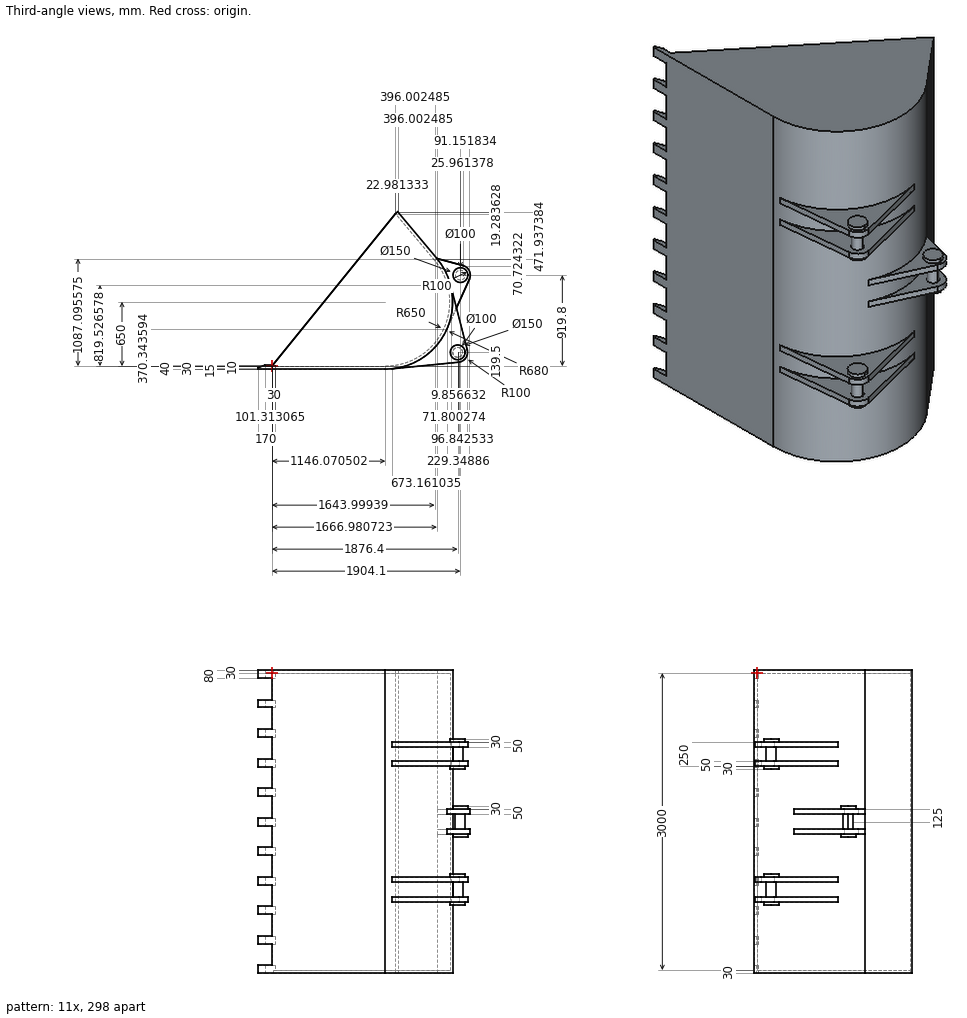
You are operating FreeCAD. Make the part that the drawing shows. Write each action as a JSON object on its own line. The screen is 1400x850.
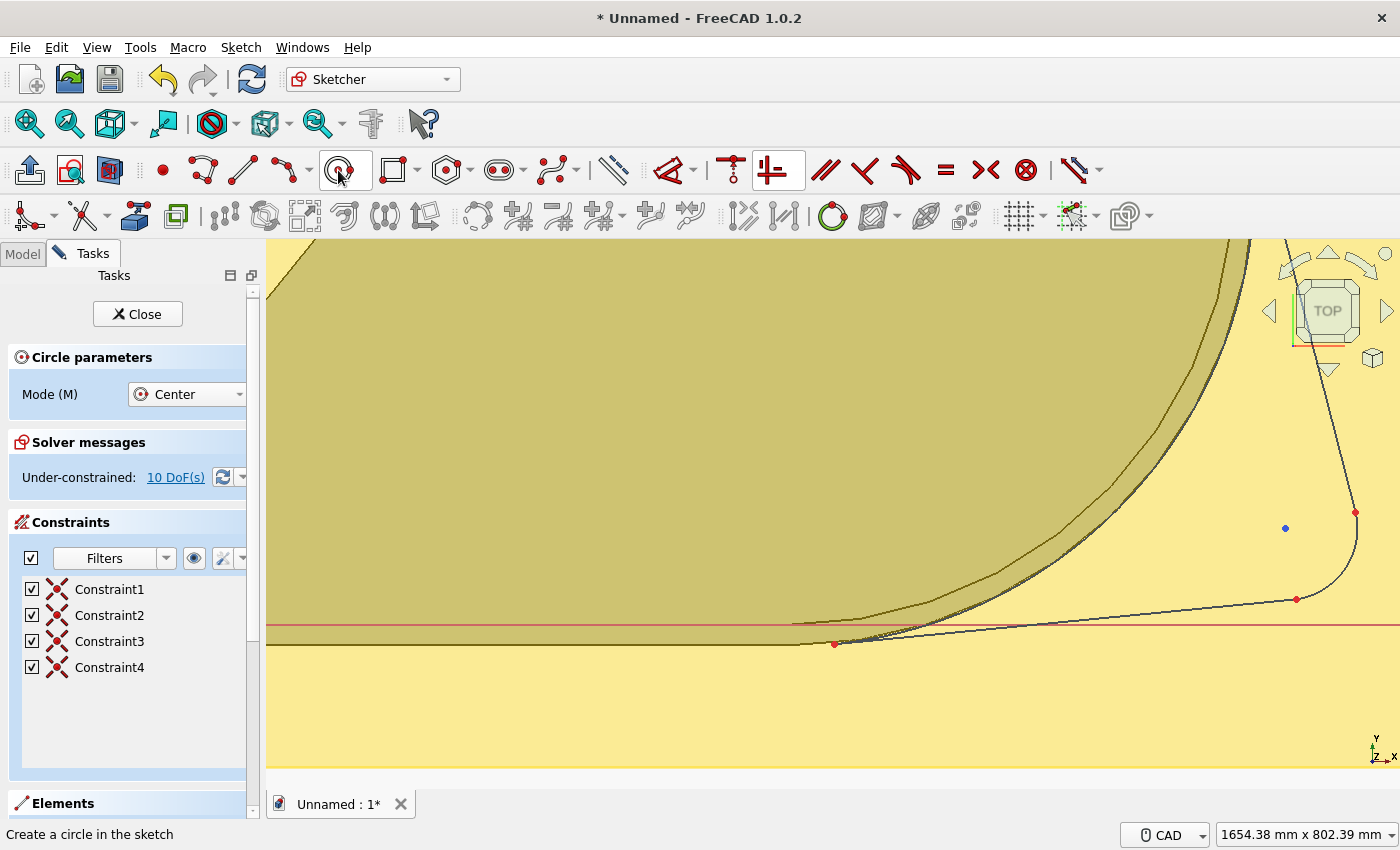
{"action": "scroll", "coordinate": [834, 645], "scroll_direction": "down", "scroll_amount": 4}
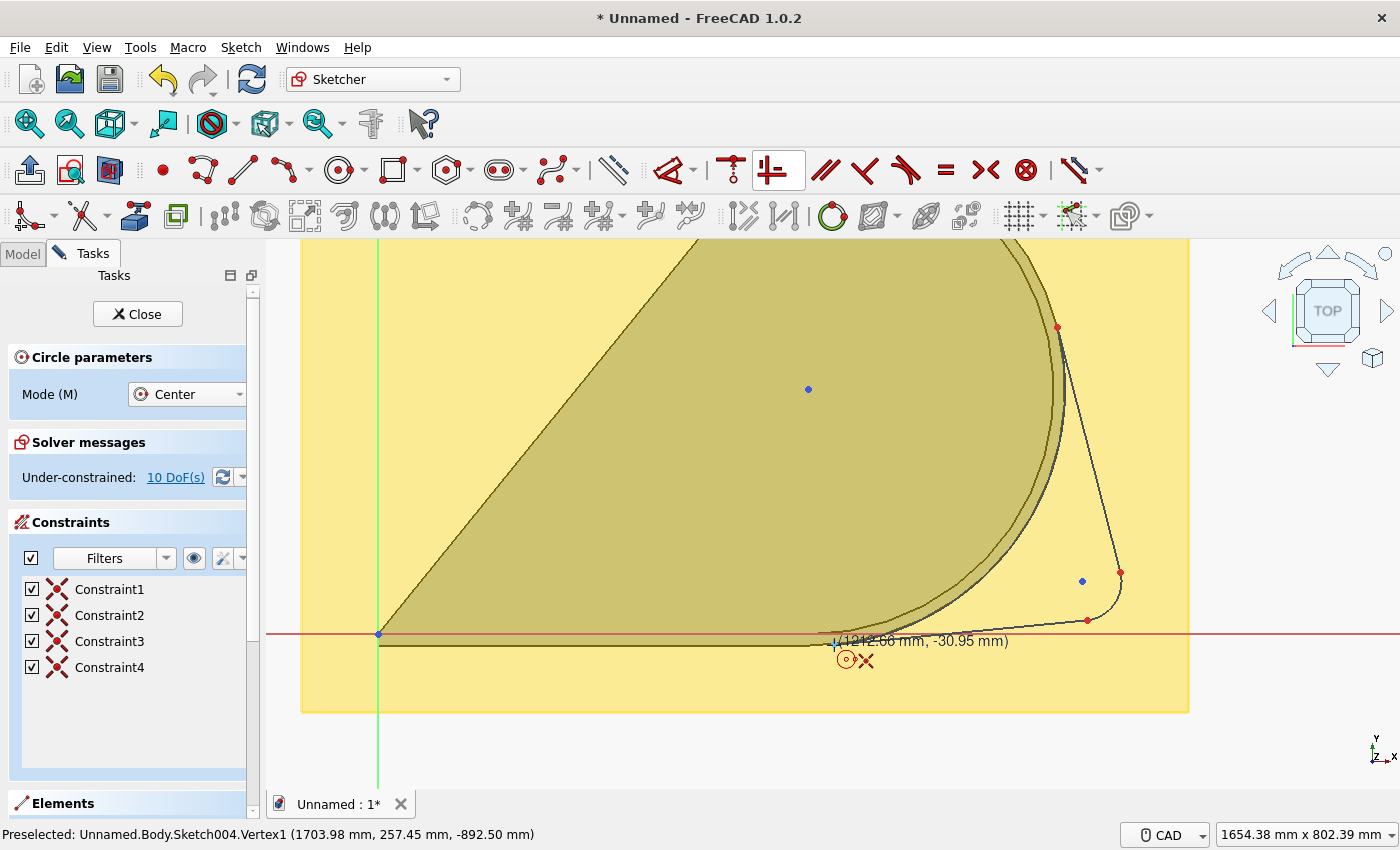
{"action": "scroll", "coordinate": [1039, 593], "scroll_direction": "up", "scroll_amount": 2}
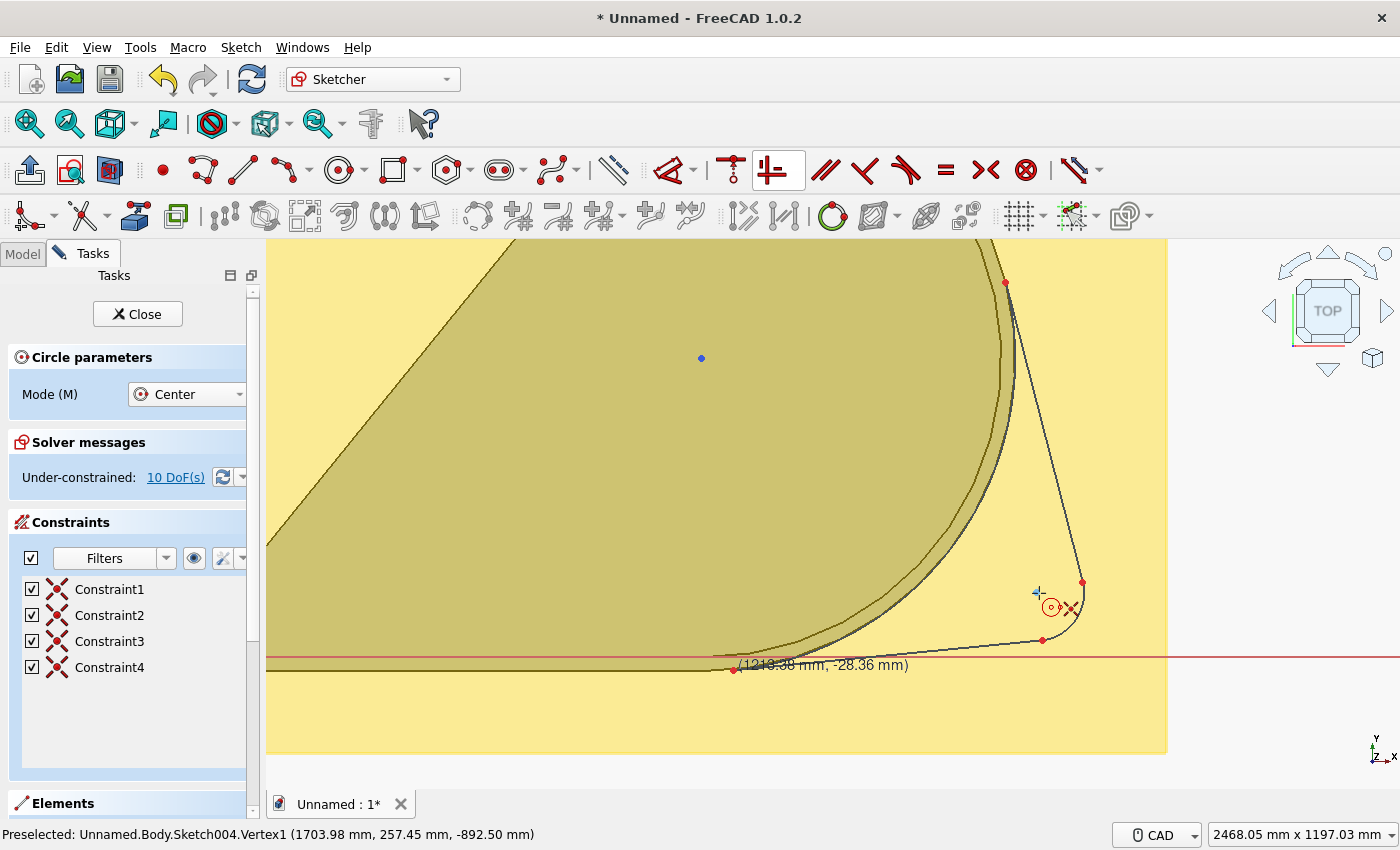
{"action": "left_click", "coordinate": [1038, 593]}
{"action": "left_click", "coordinate": [1054, 577]}
{"action": "key", "text": "Escape"}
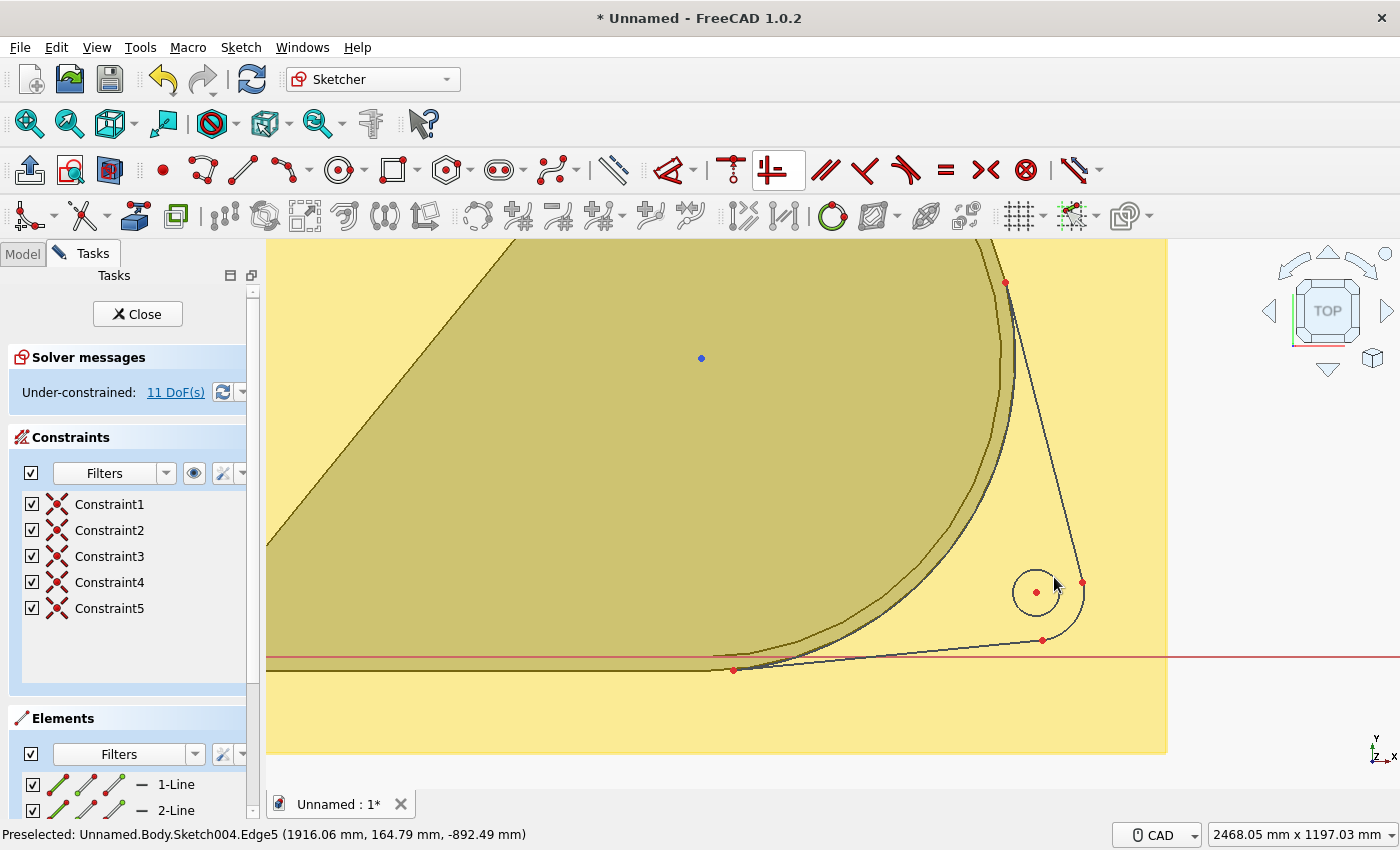
{"action": "key", "text": "d"}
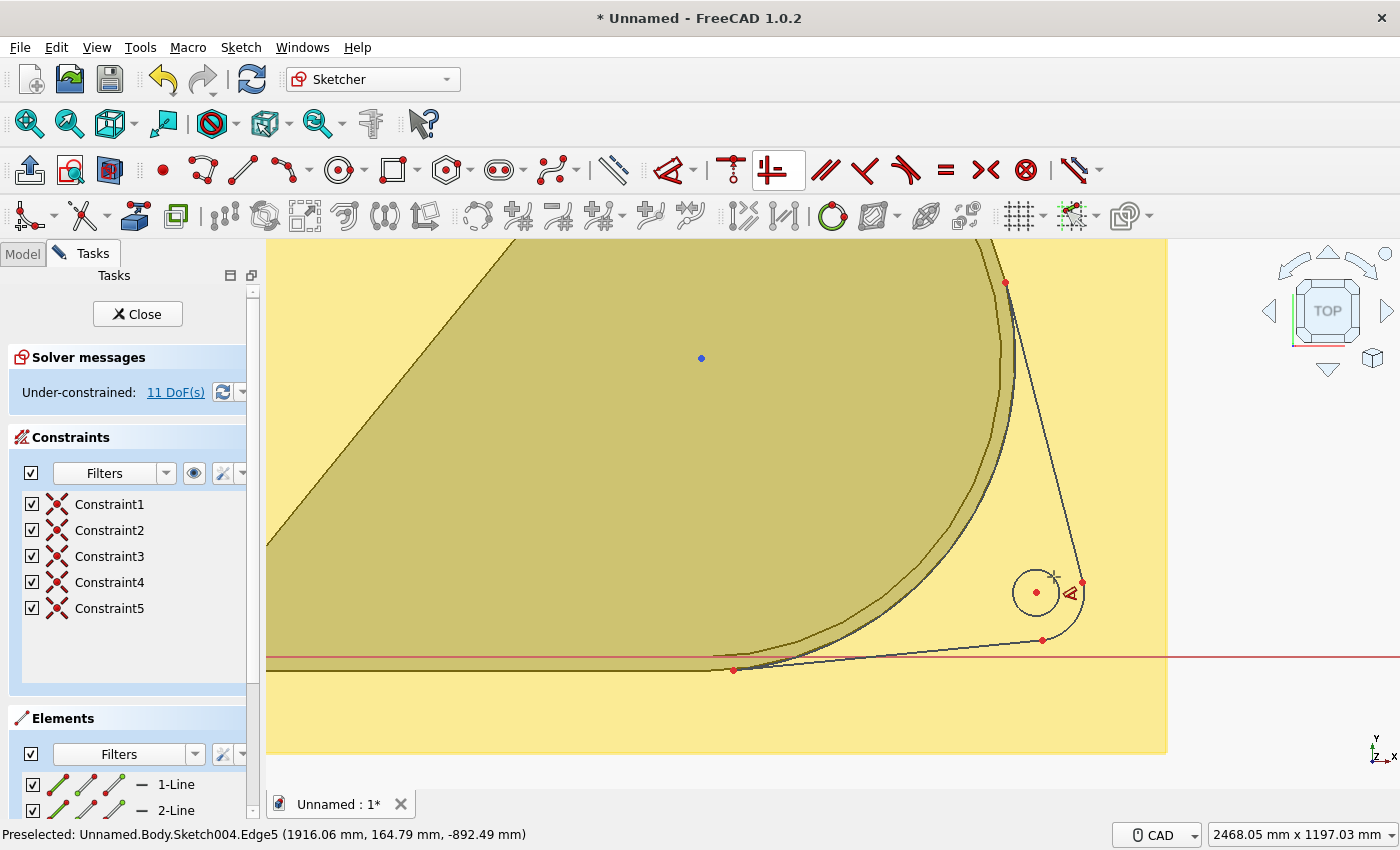
{"action": "left_click", "coordinate": [1065, 631]}
{"action": "left_click", "coordinate": [1048, 672]}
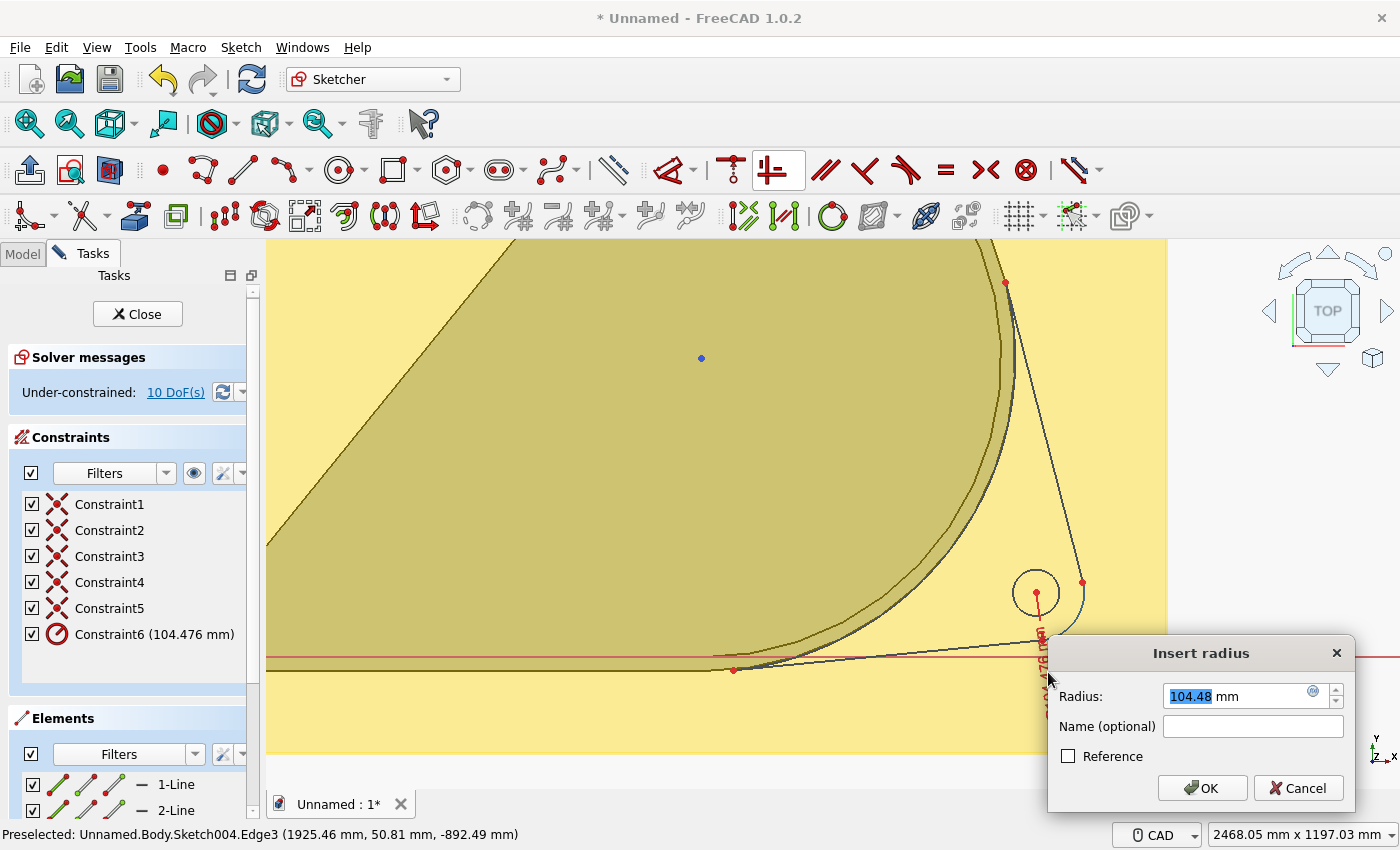
{"action": "type", "text": "100"}
{"action": "key", "text": "Return"}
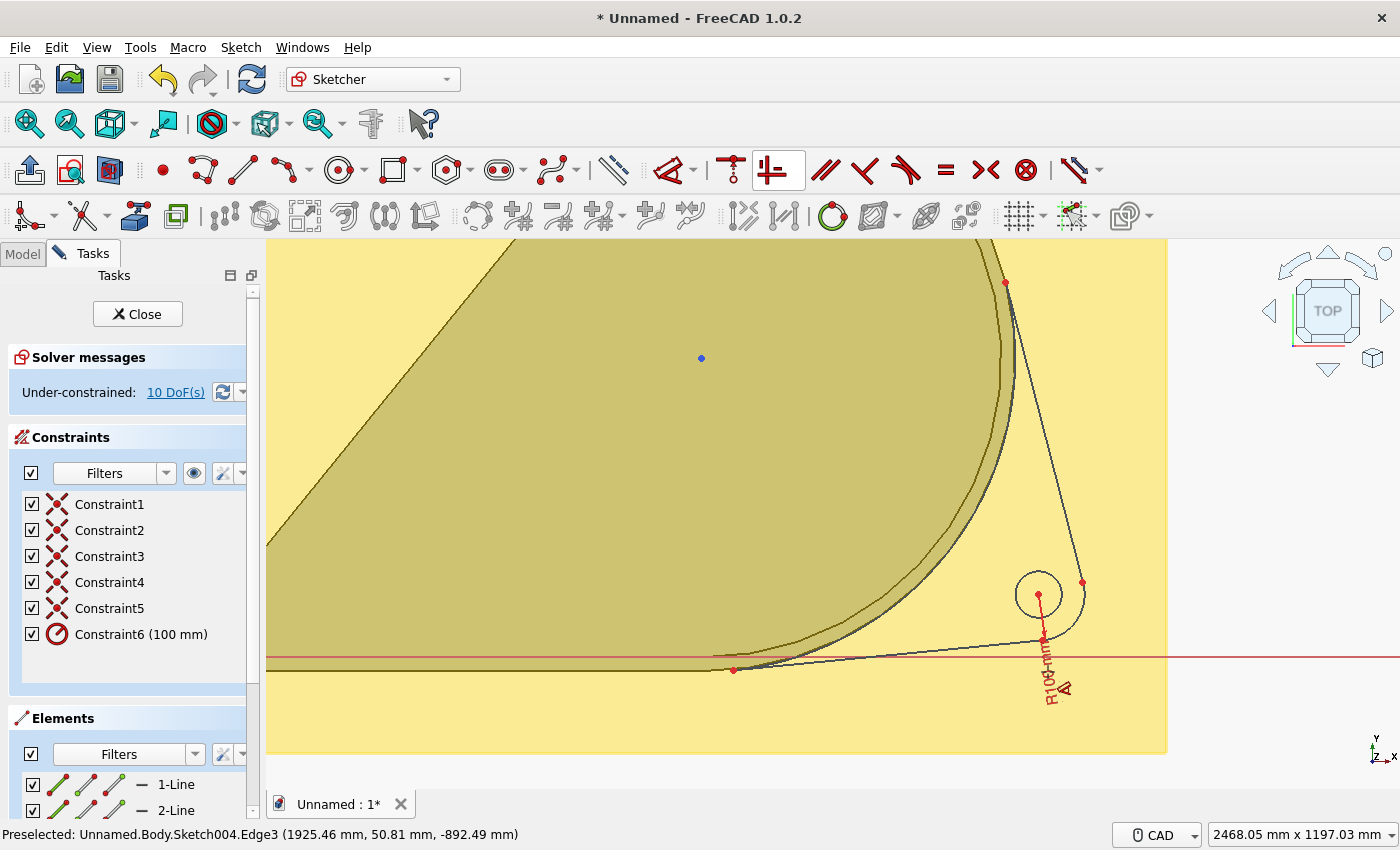
{"action": "left_click", "coordinate": [883, 614]}
{"action": "left_click", "coordinate": [902, 640]}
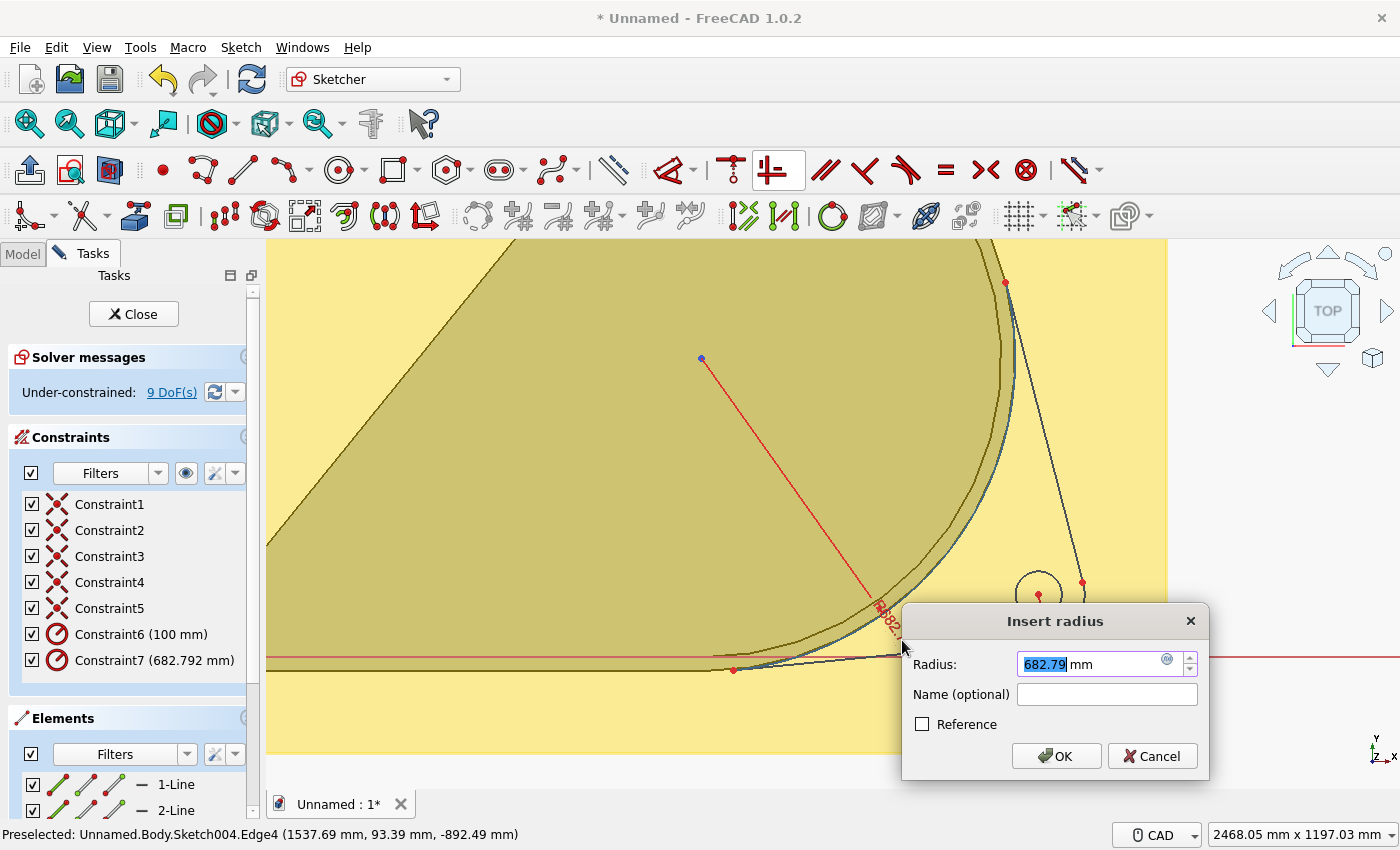
{"action": "type", "text": "680"}
{"action": "key", "text": "Return"}